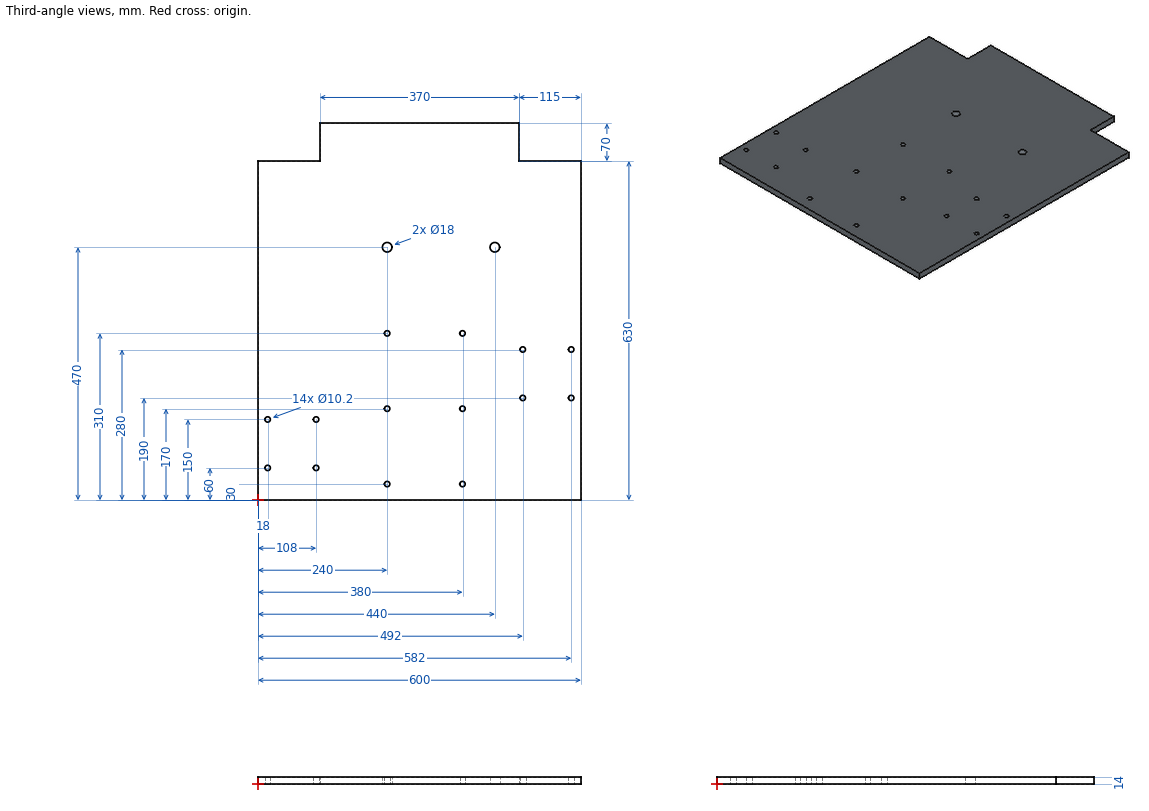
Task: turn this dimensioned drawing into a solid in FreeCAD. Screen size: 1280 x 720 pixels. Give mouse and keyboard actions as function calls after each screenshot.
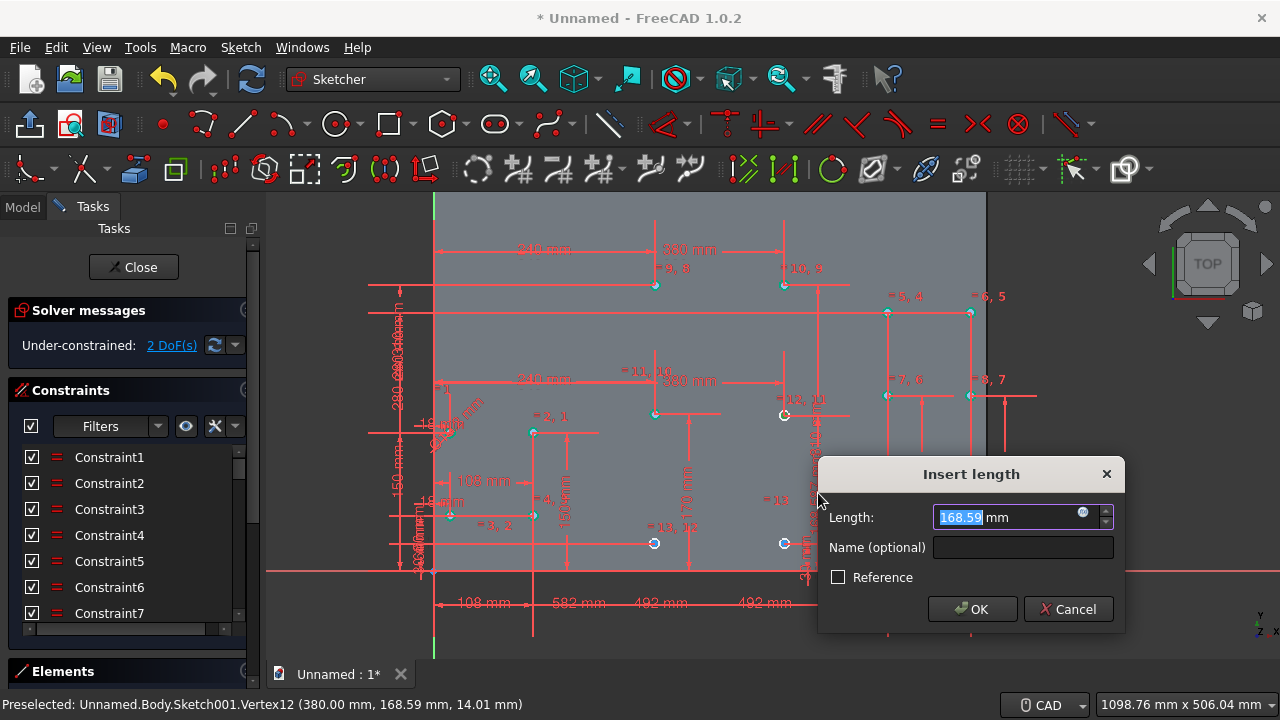
text(170)
key(Return)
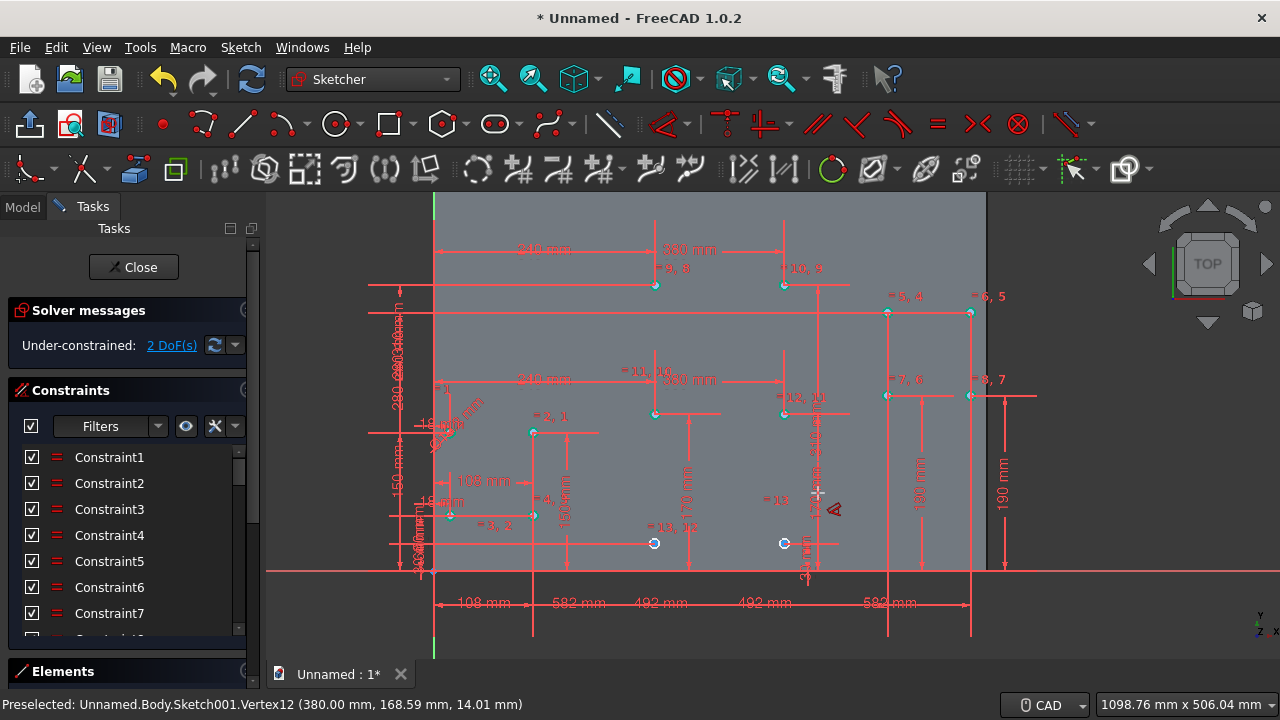
click(655, 544)
click(544, 629)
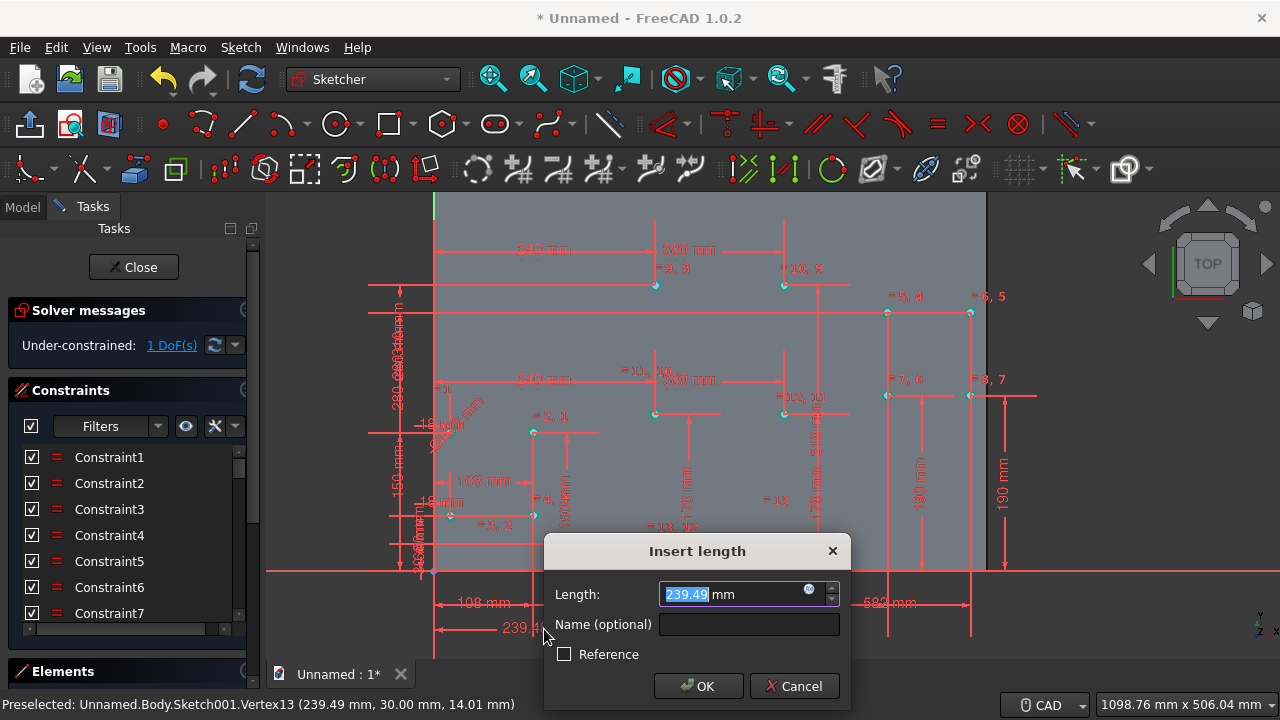
text(240)
key(Return)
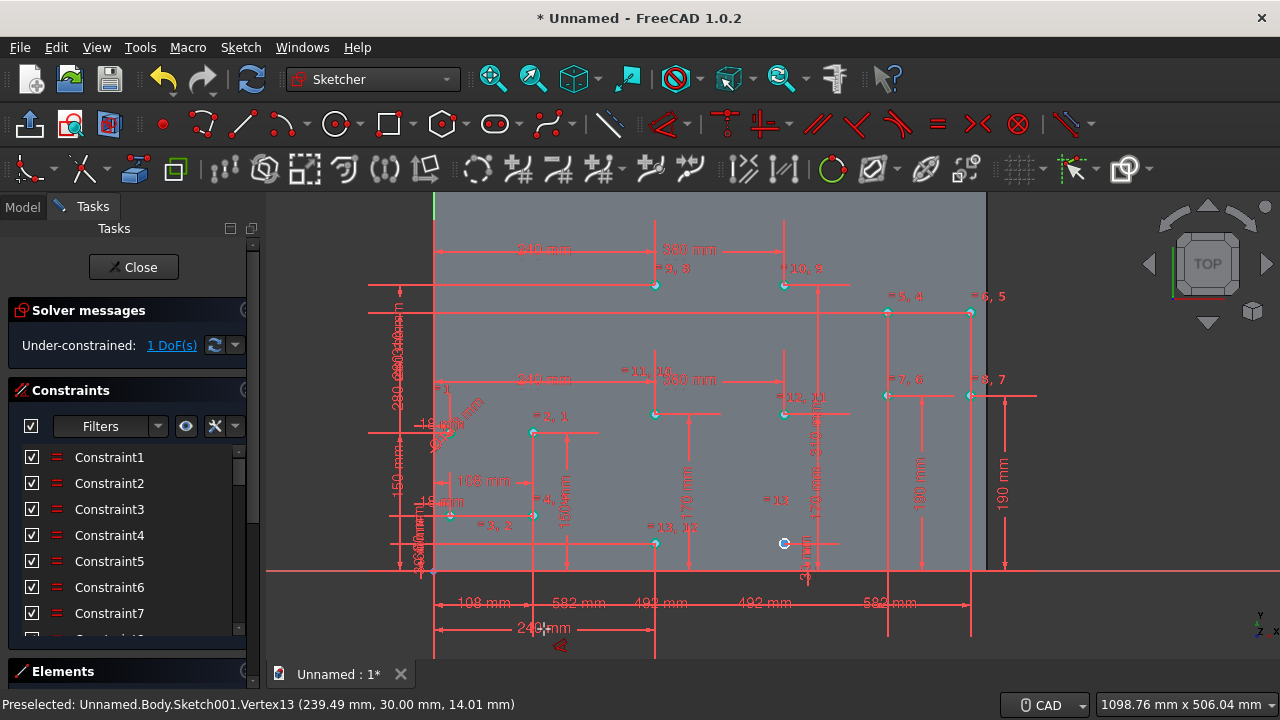
click(785, 544)
click(690, 629)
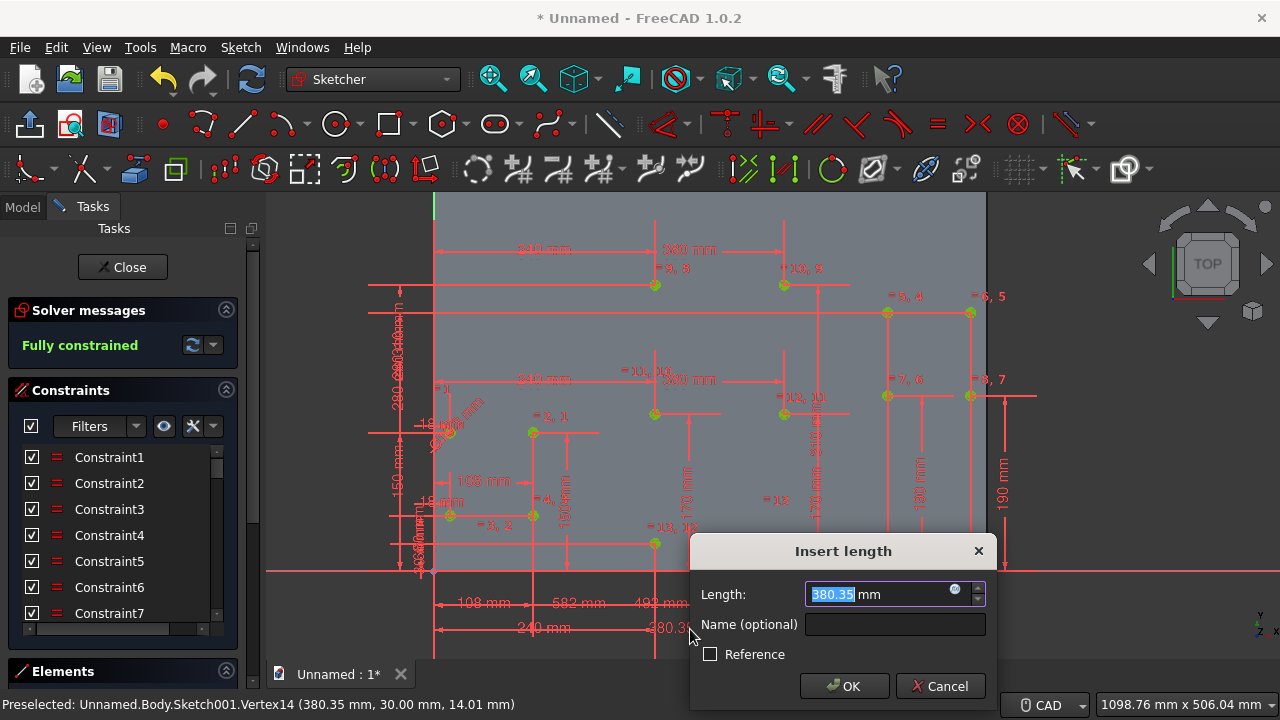
text(380)
key(Return)
key(Escape)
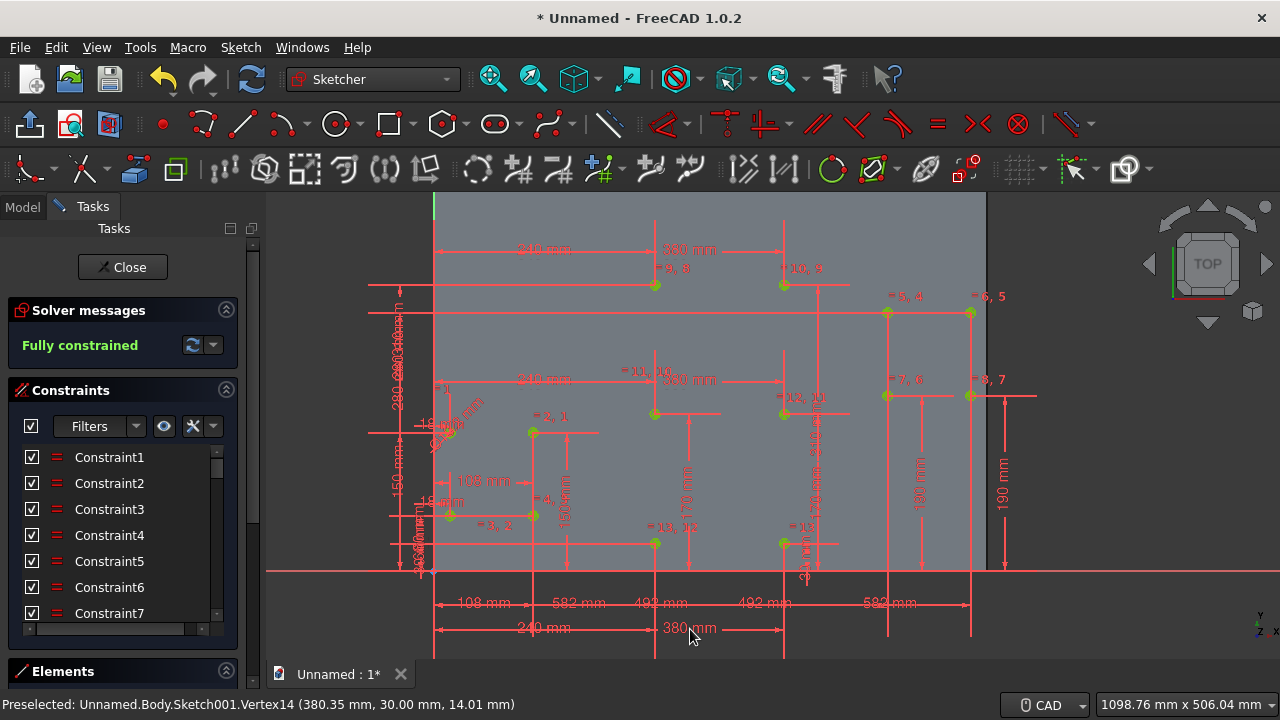
click(123, 267)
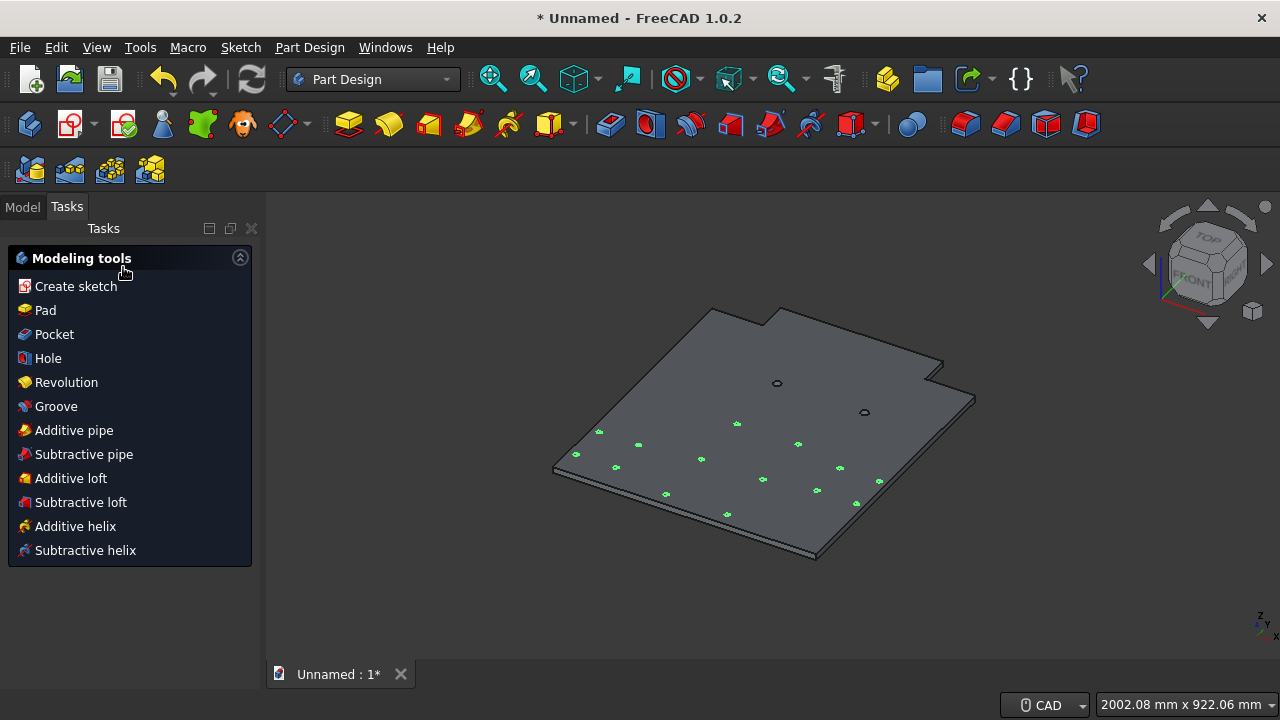
click(612, 124)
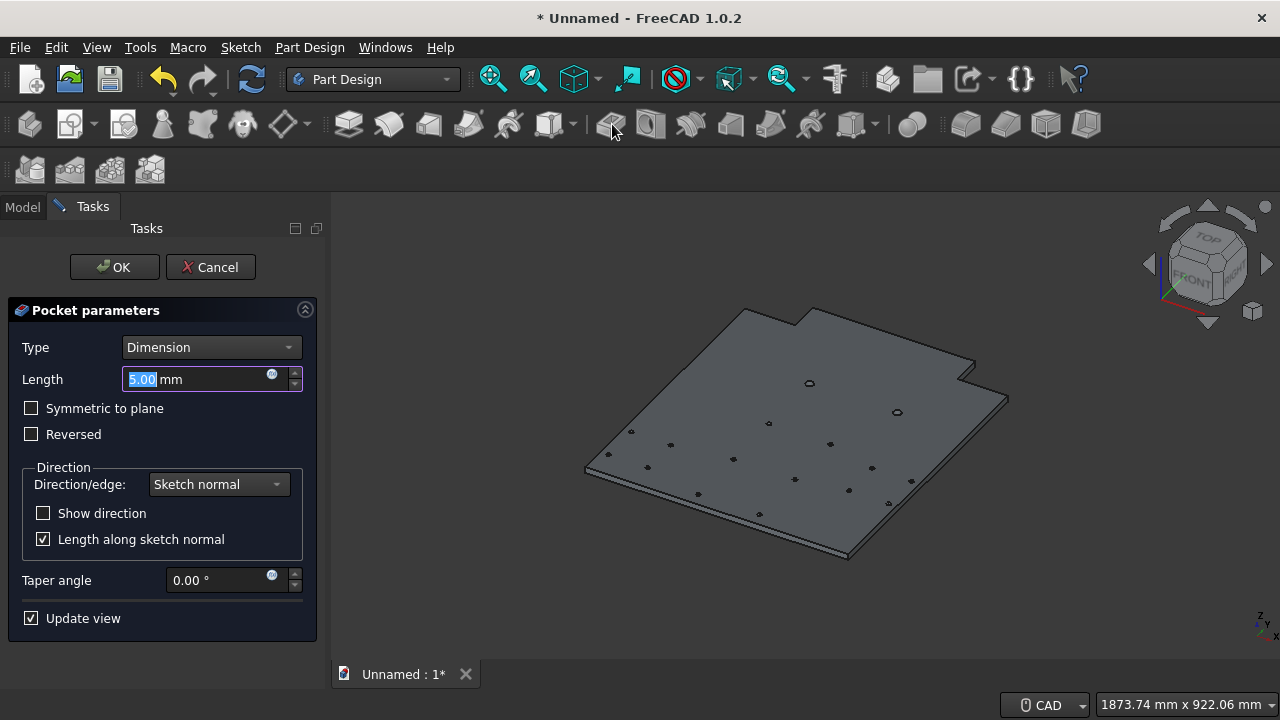
click(212, 348)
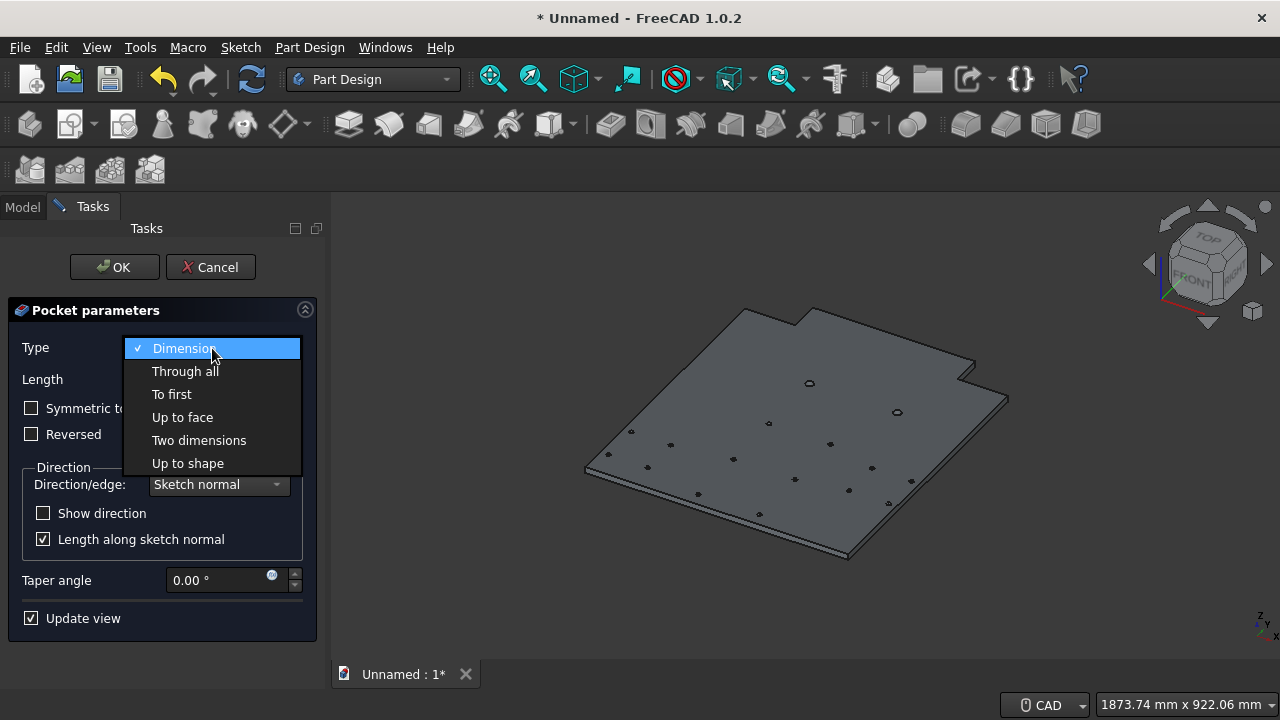
click(212, 372)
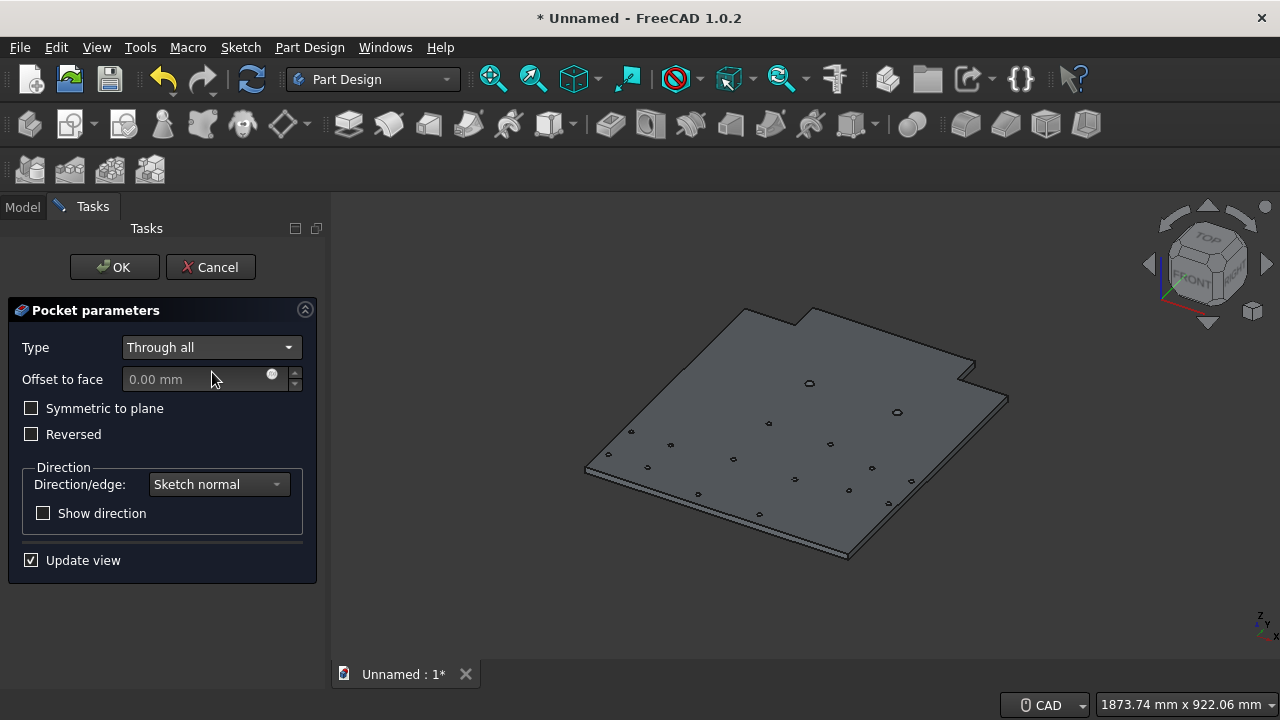
click(115, 267)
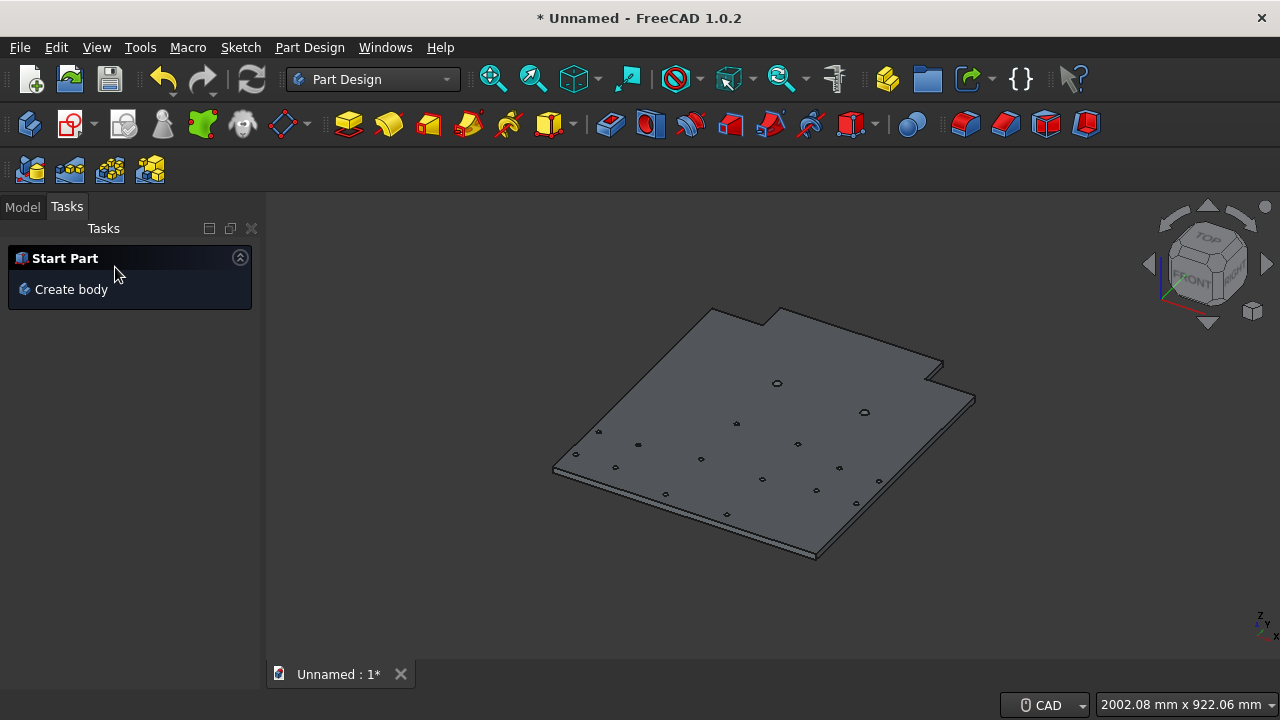
key(0)